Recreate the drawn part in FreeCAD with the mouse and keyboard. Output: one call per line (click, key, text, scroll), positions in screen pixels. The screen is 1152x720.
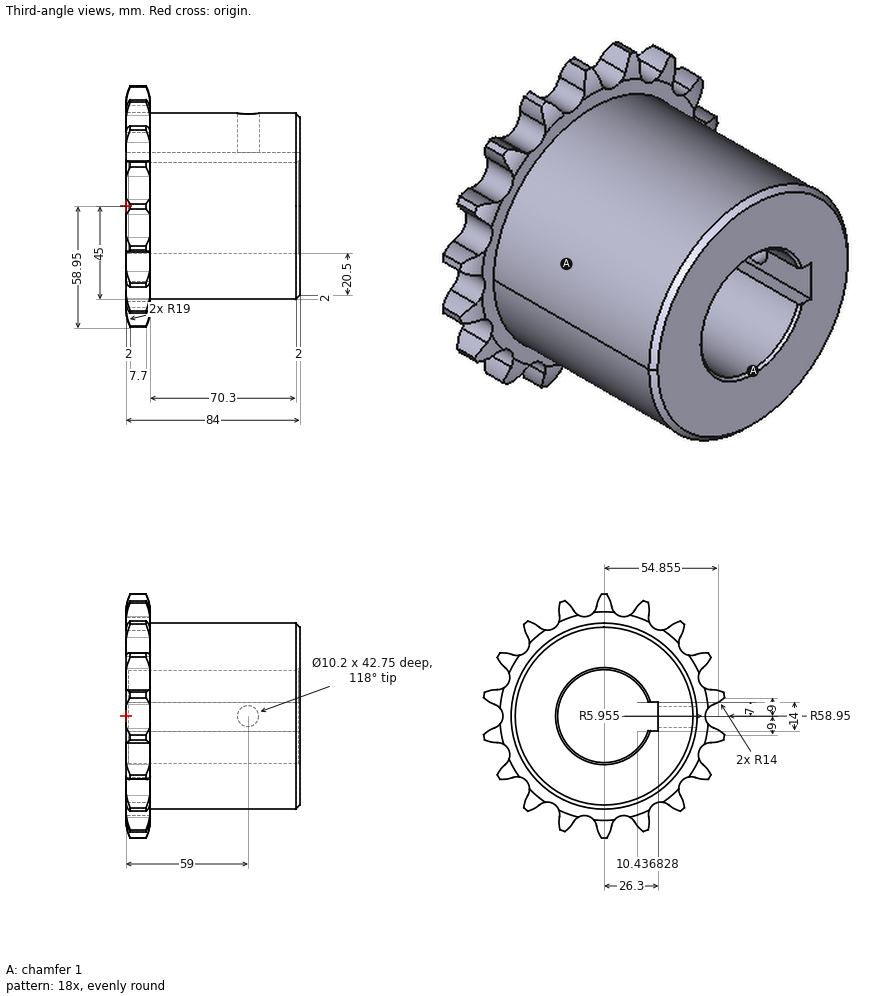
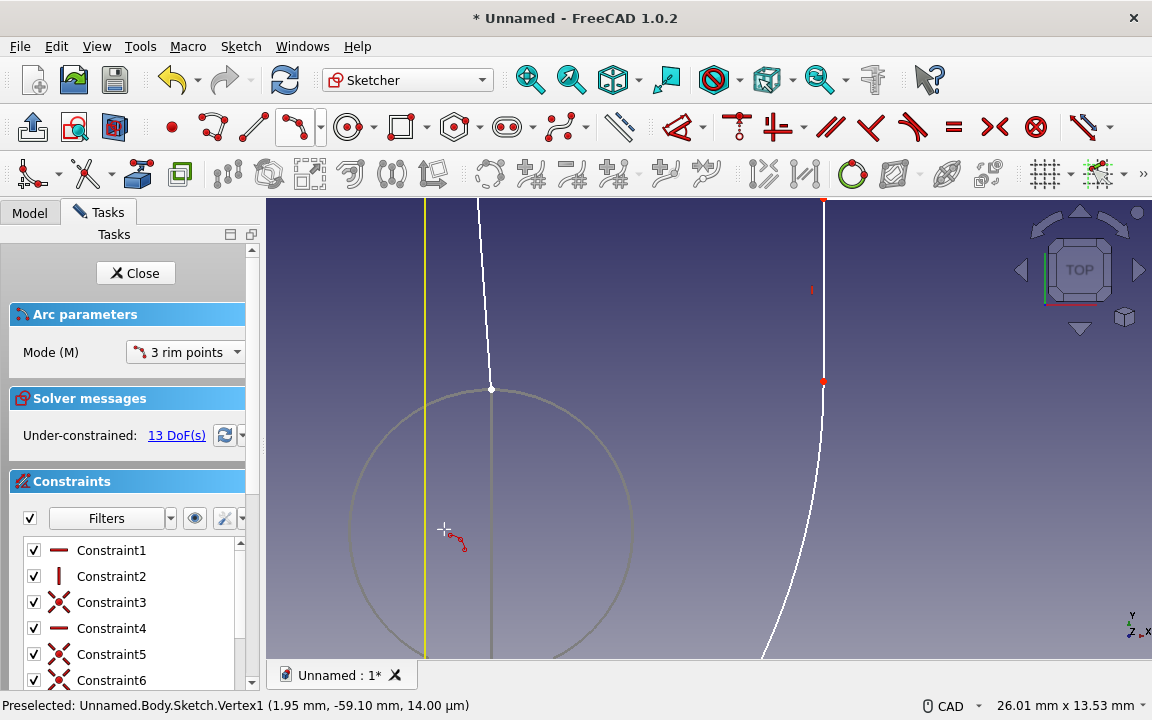
click(442, 528)
key(Escape)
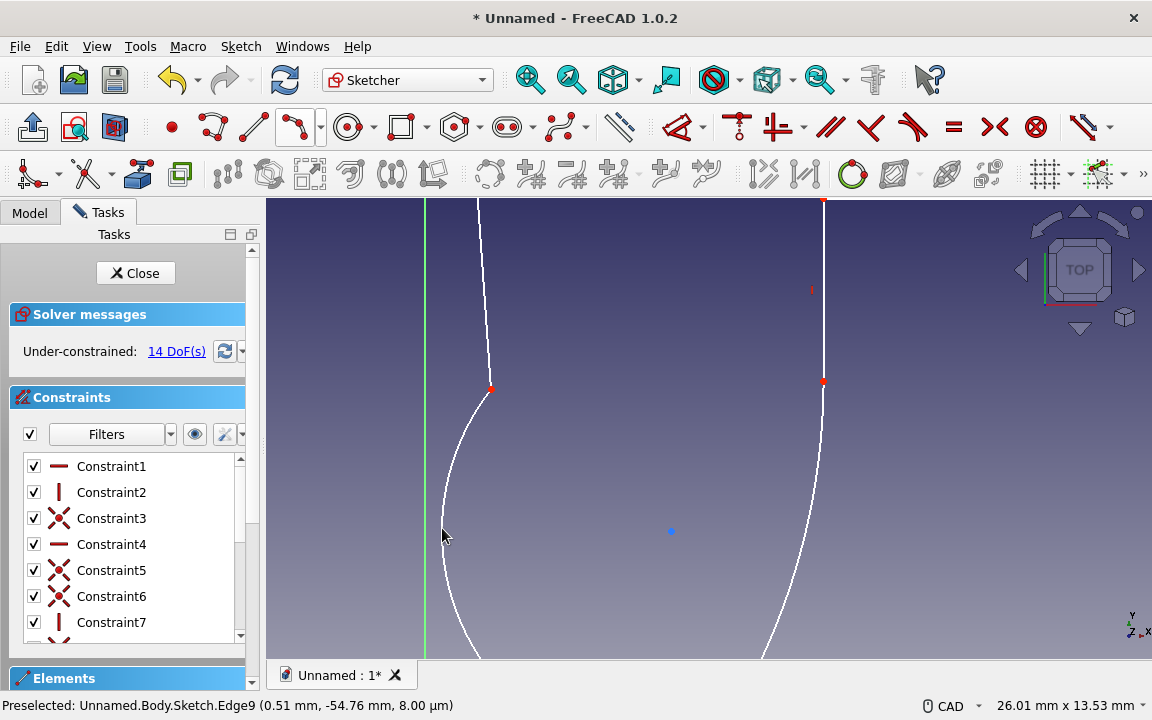
scroll(450, 548, down, 10)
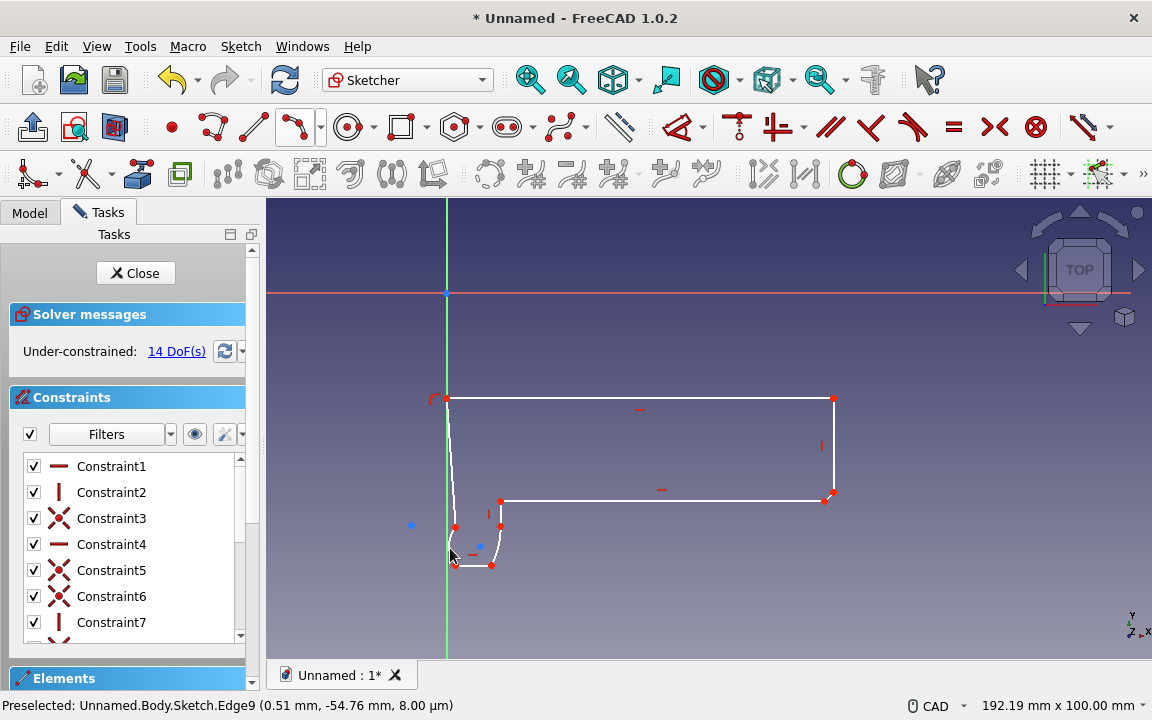
scroll(501, 519, up, 4)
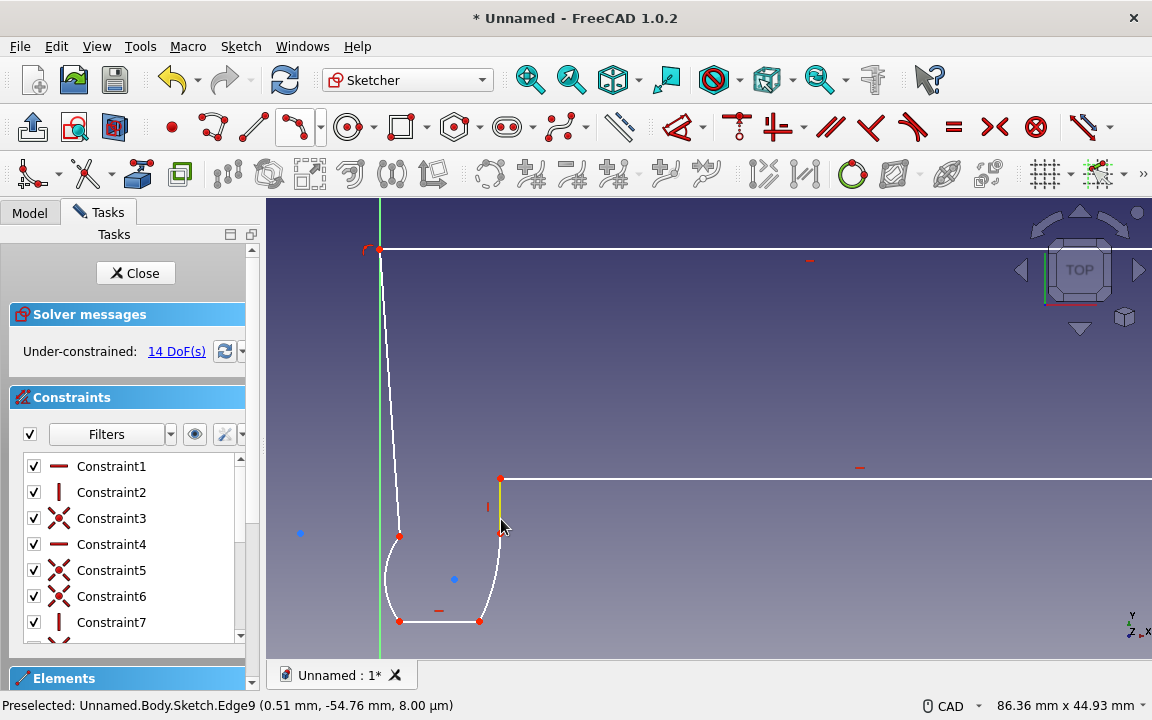
click(500, 517)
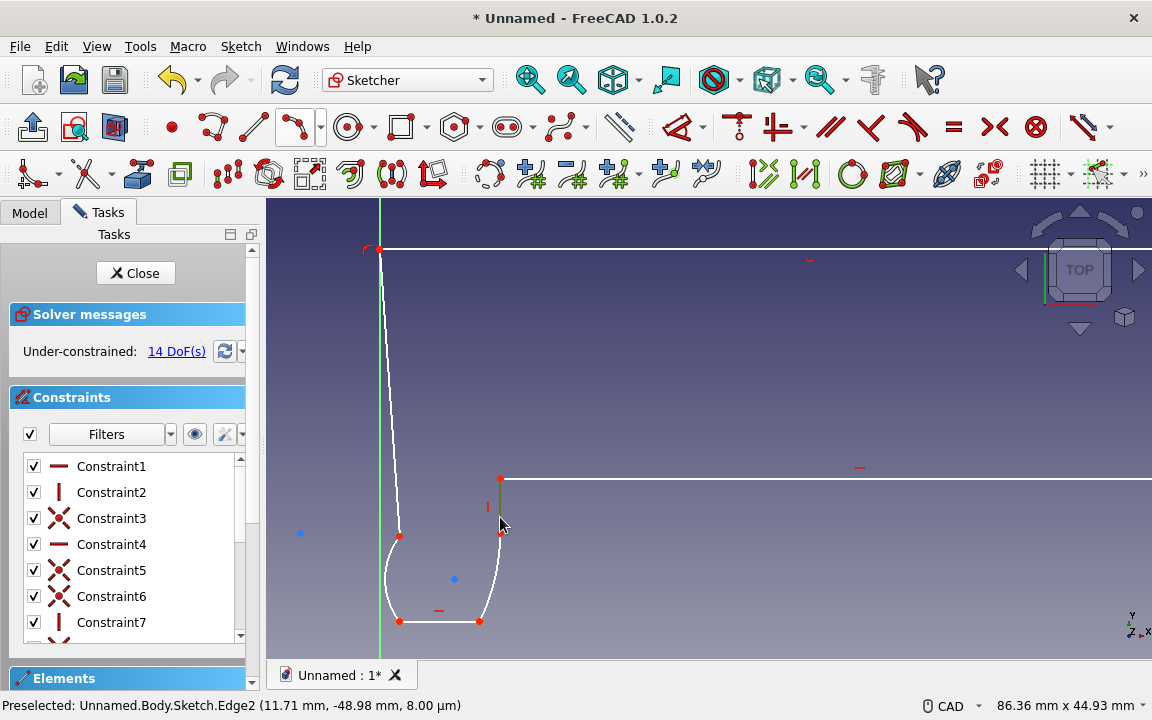
click(490, 597)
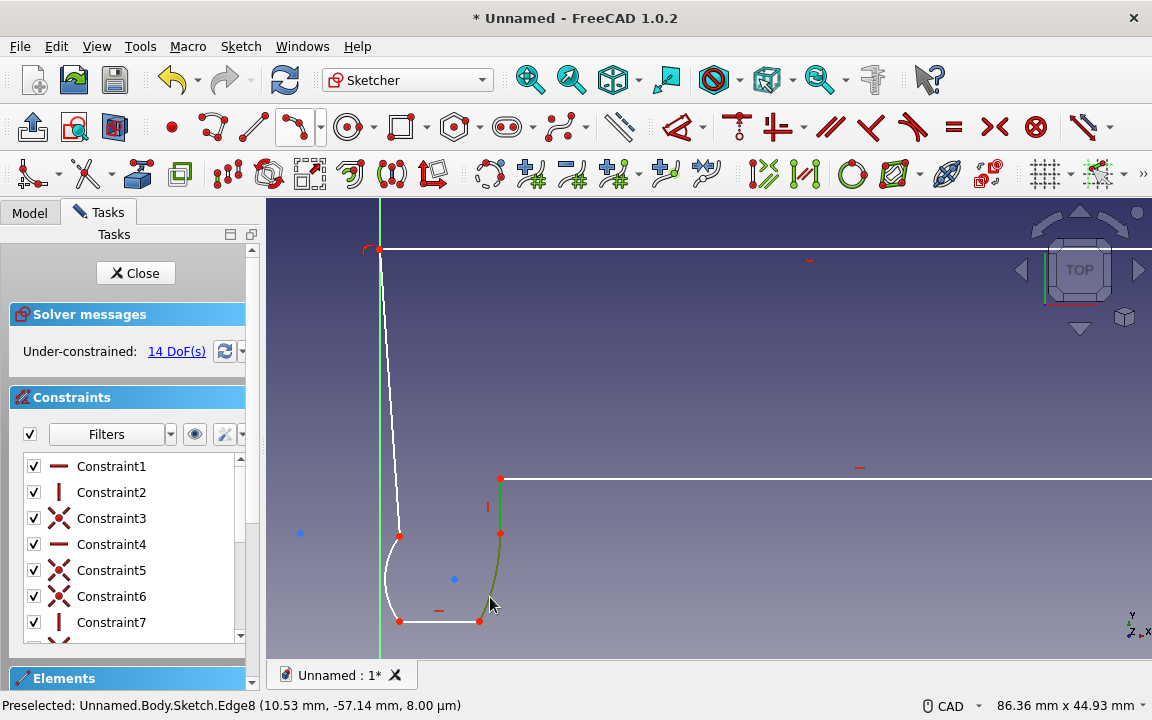
click(913, 128)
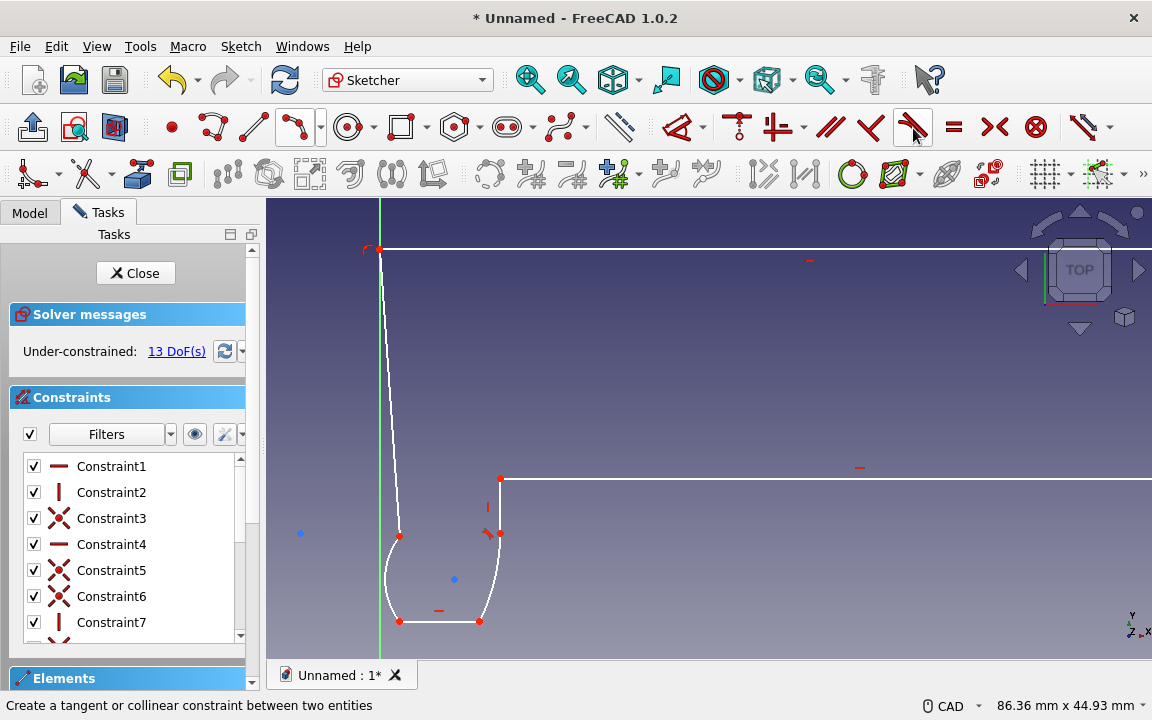
click(394, 450)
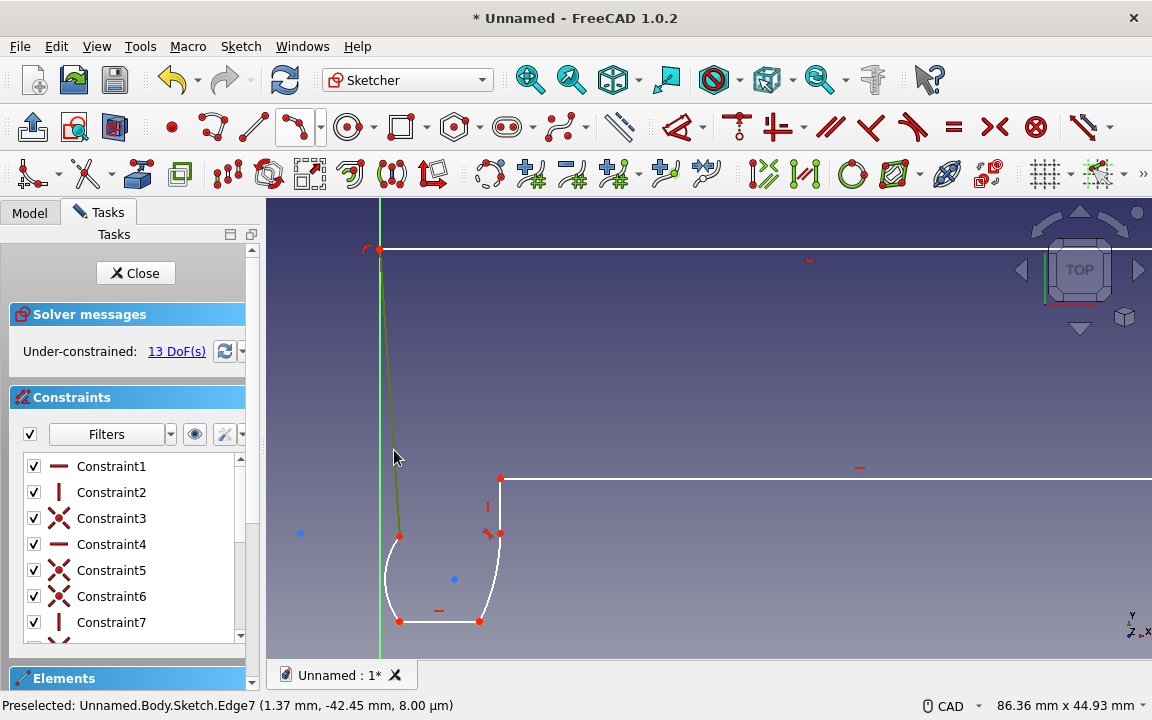
scroll(391, 552, up, 2)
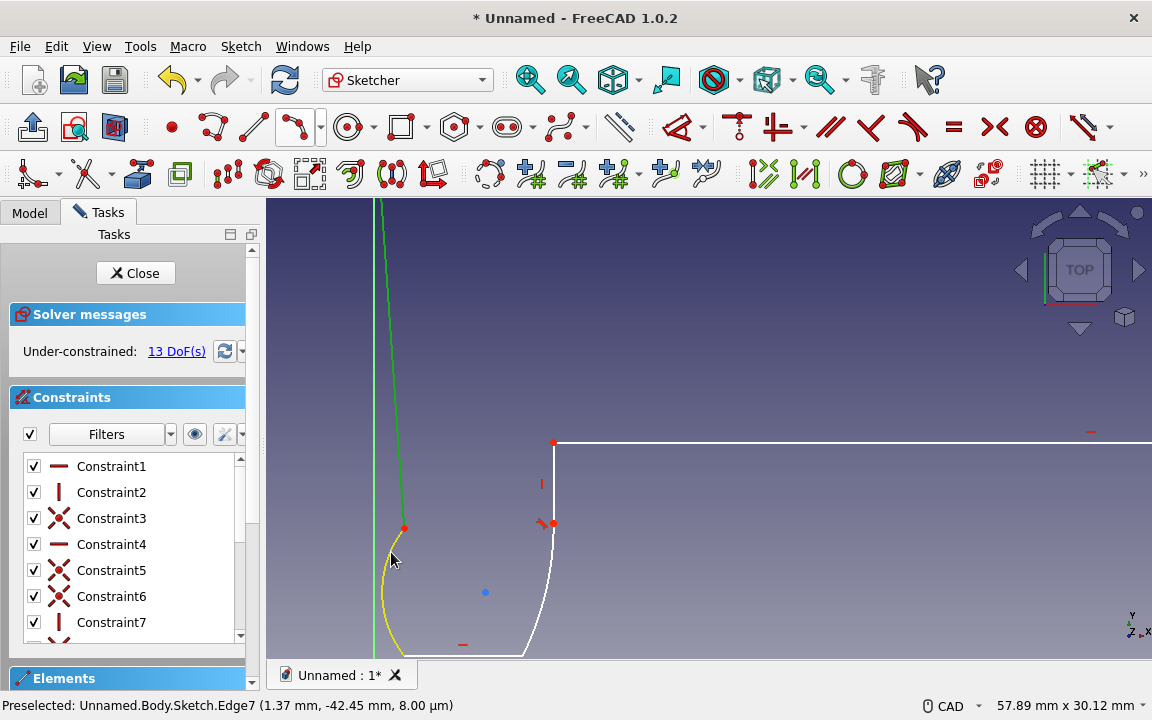
click(390, 552)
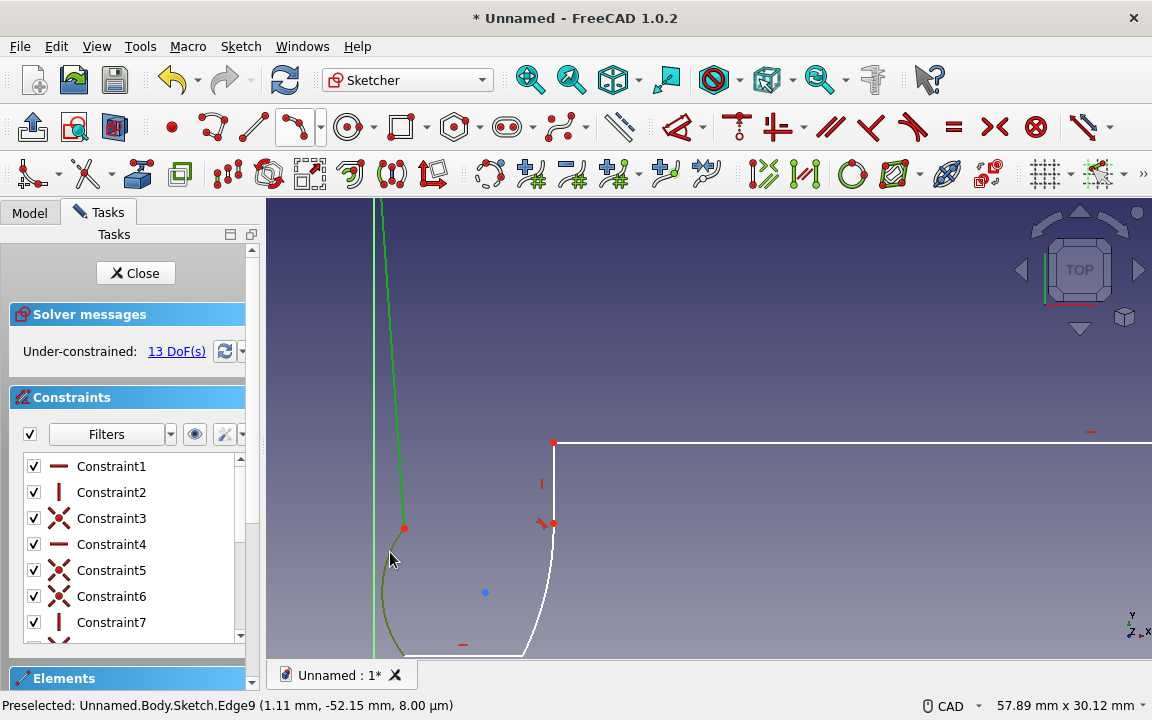
click(913, 128)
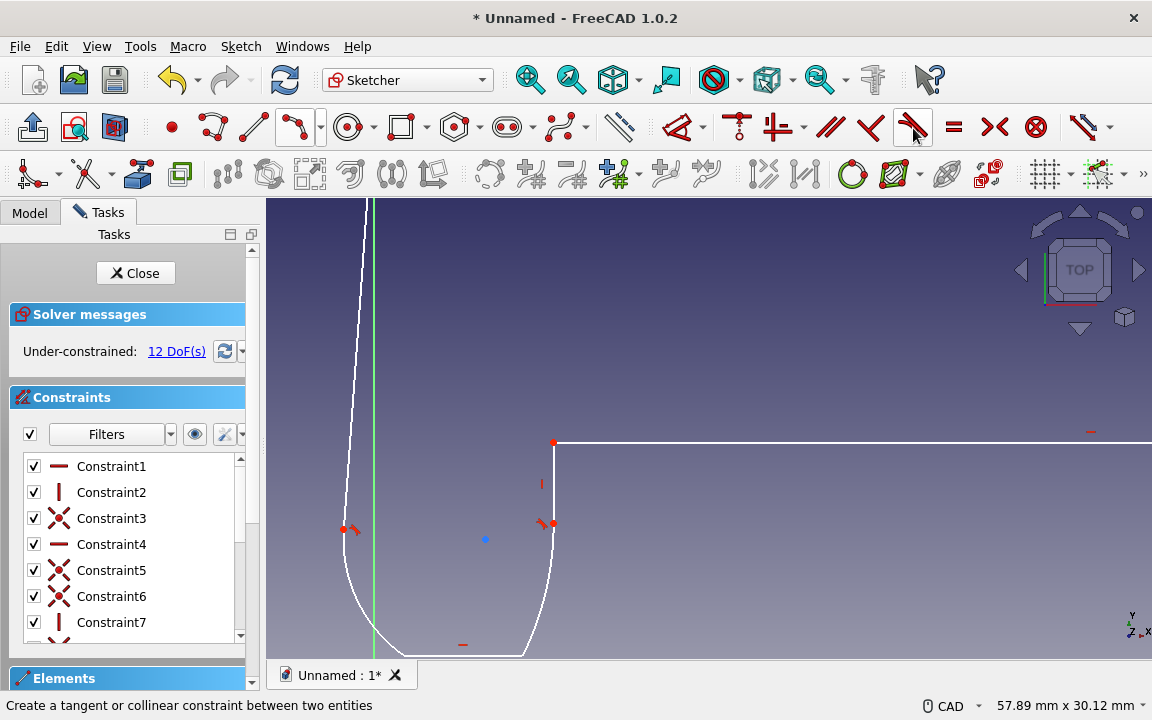
scroll(365, 229, up, 3)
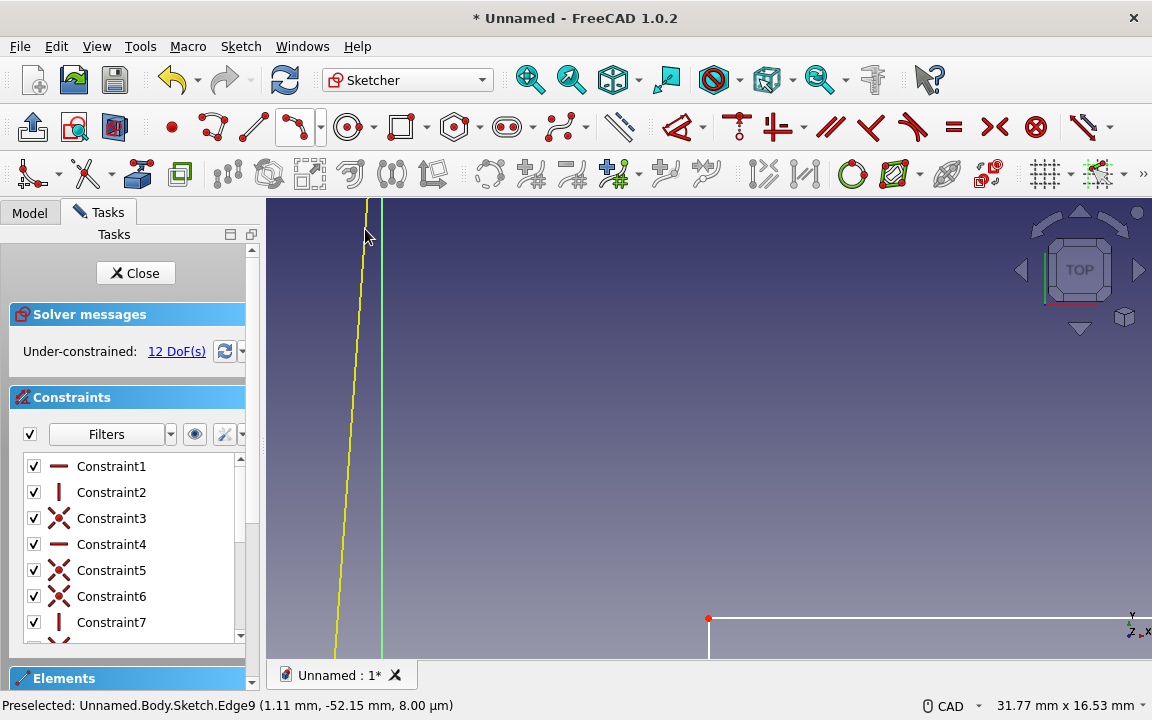
click(365, 229)